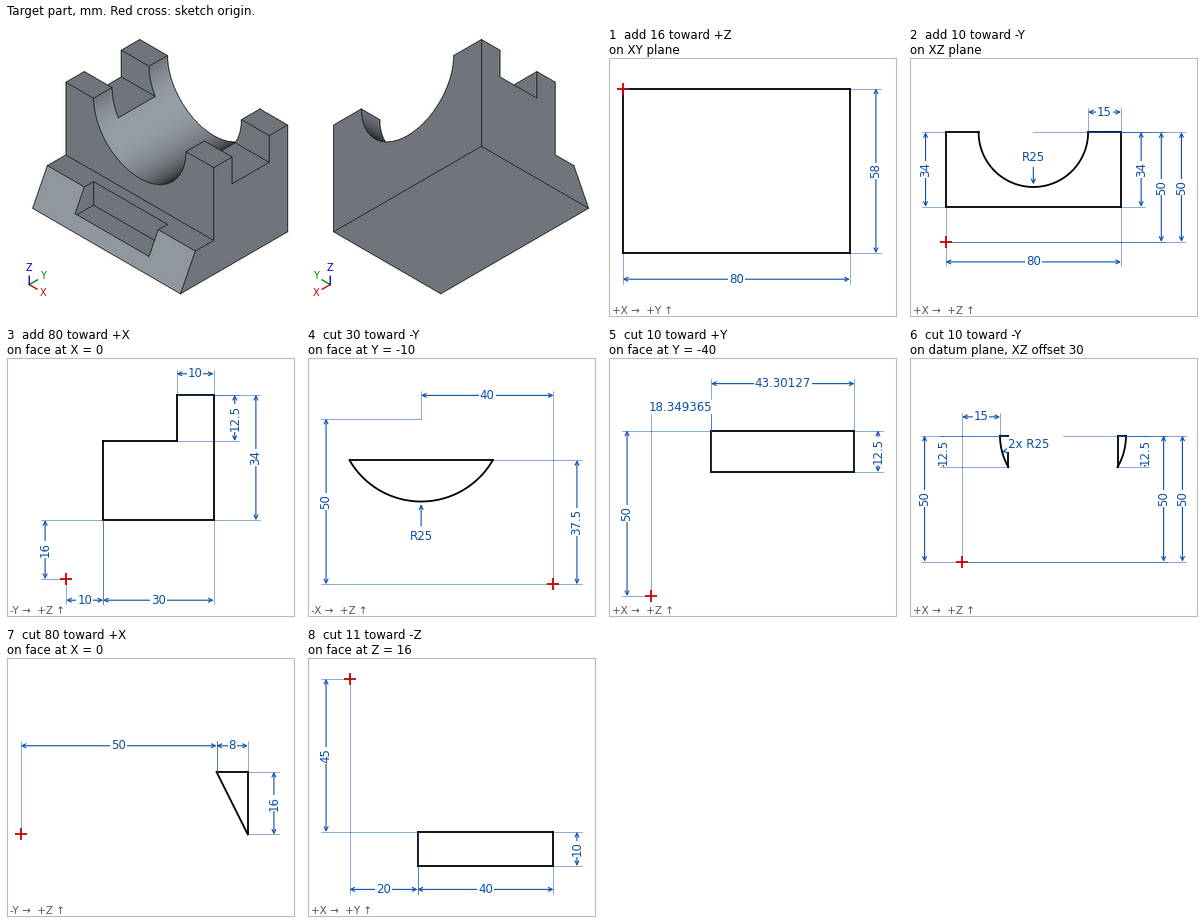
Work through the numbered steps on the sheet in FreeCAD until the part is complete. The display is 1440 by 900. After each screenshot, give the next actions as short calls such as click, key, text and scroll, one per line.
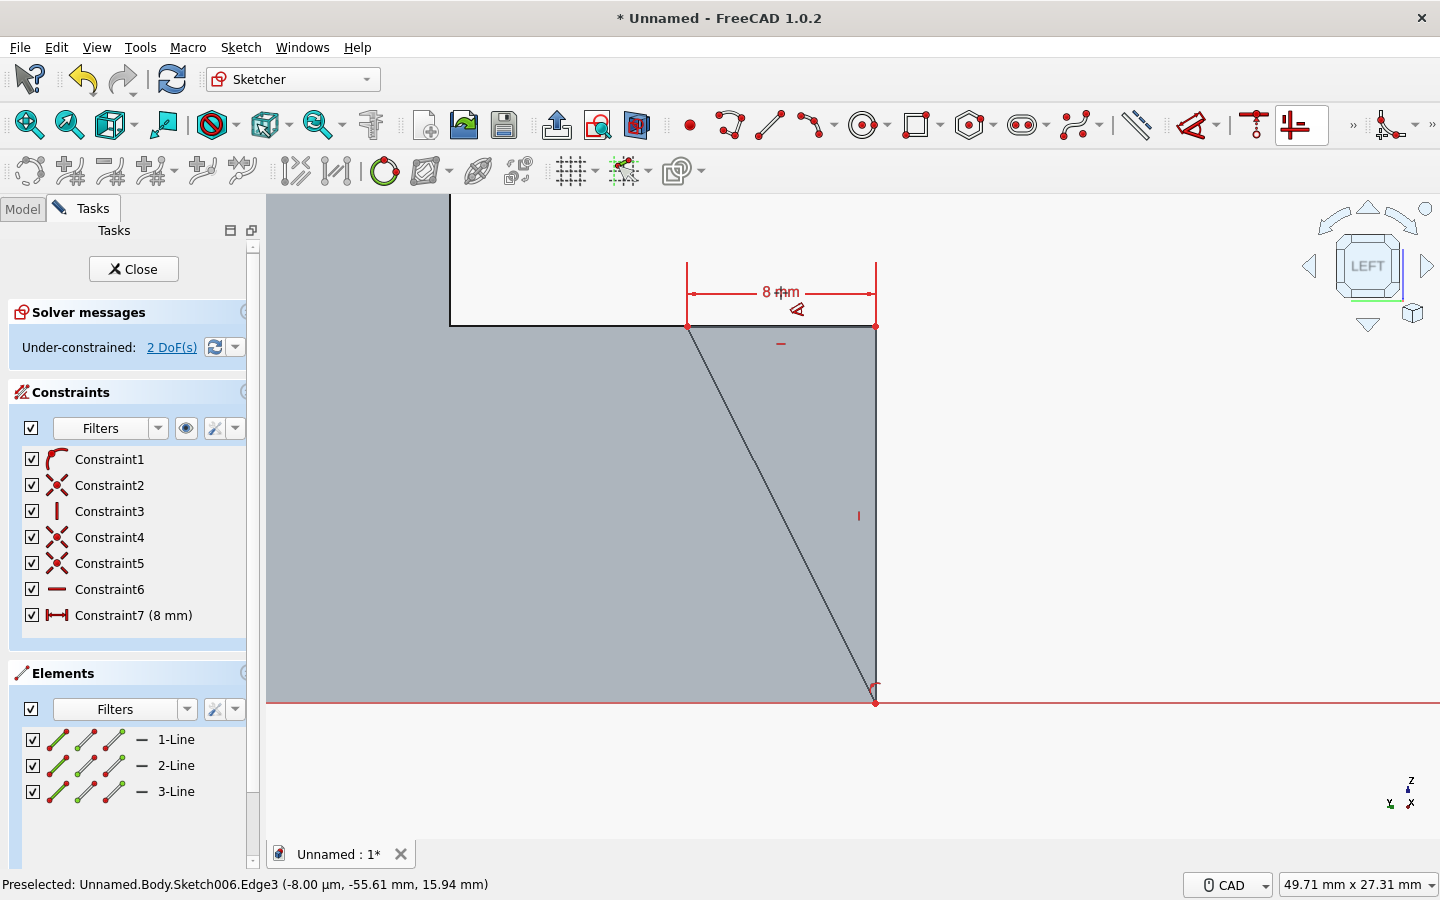
click(876, 591)
click(910, 515)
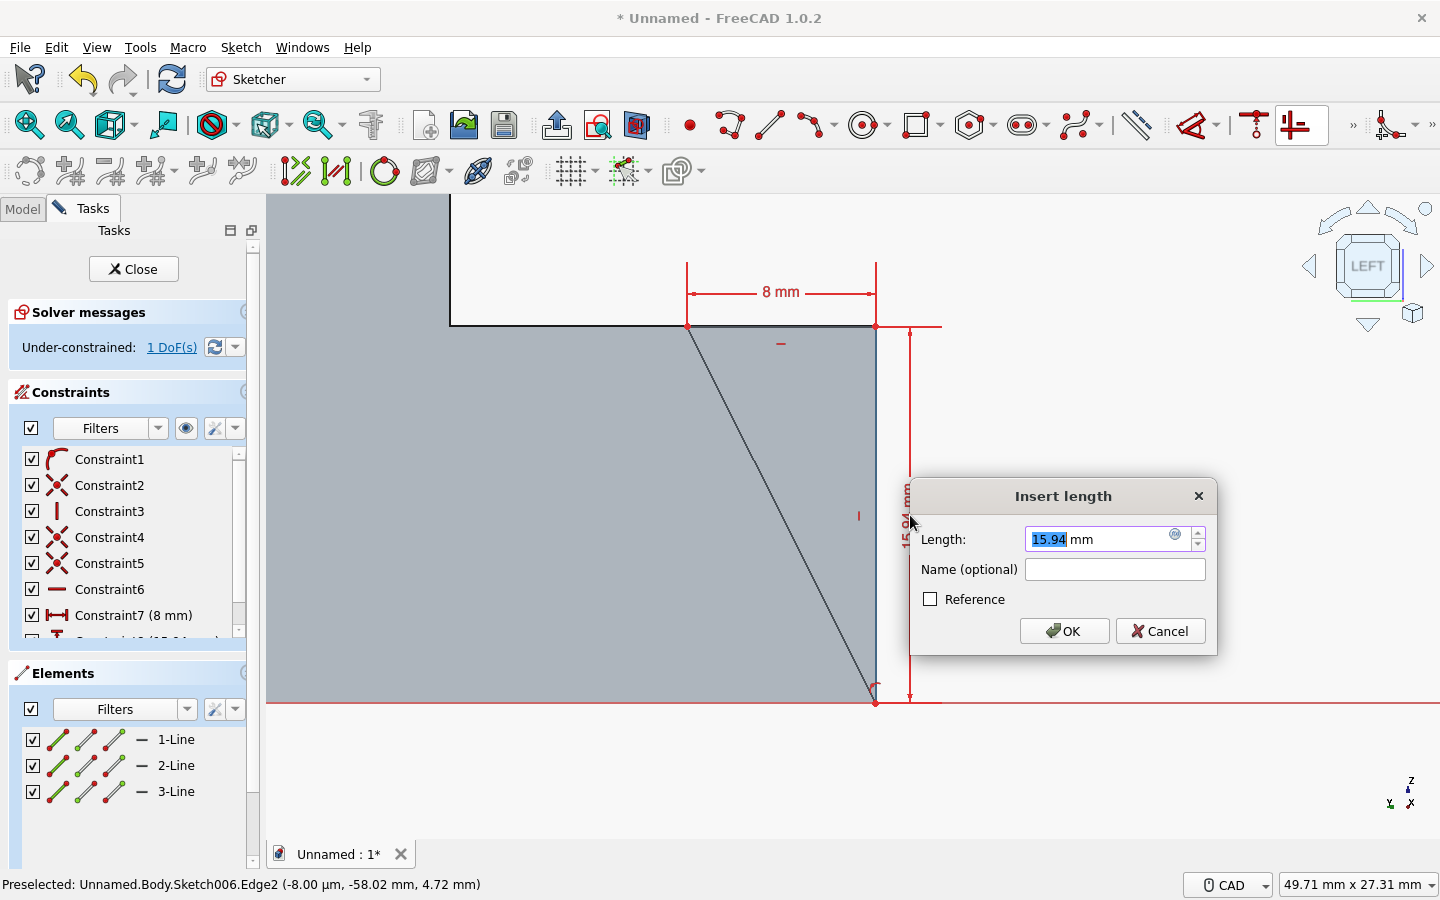
text(16)
key(Return)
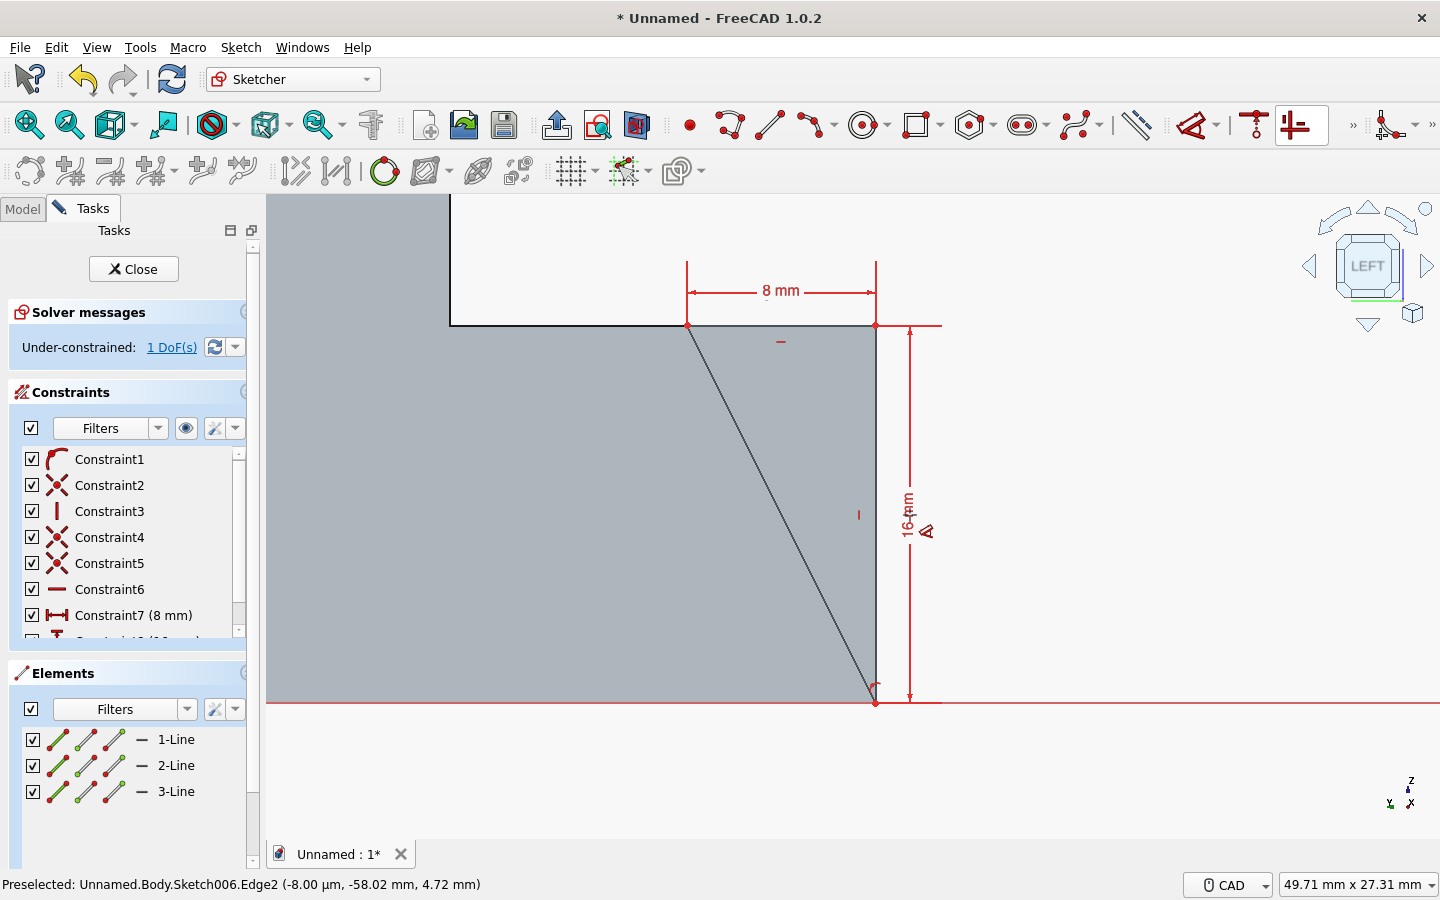
click(687, 326)
click(490, 737)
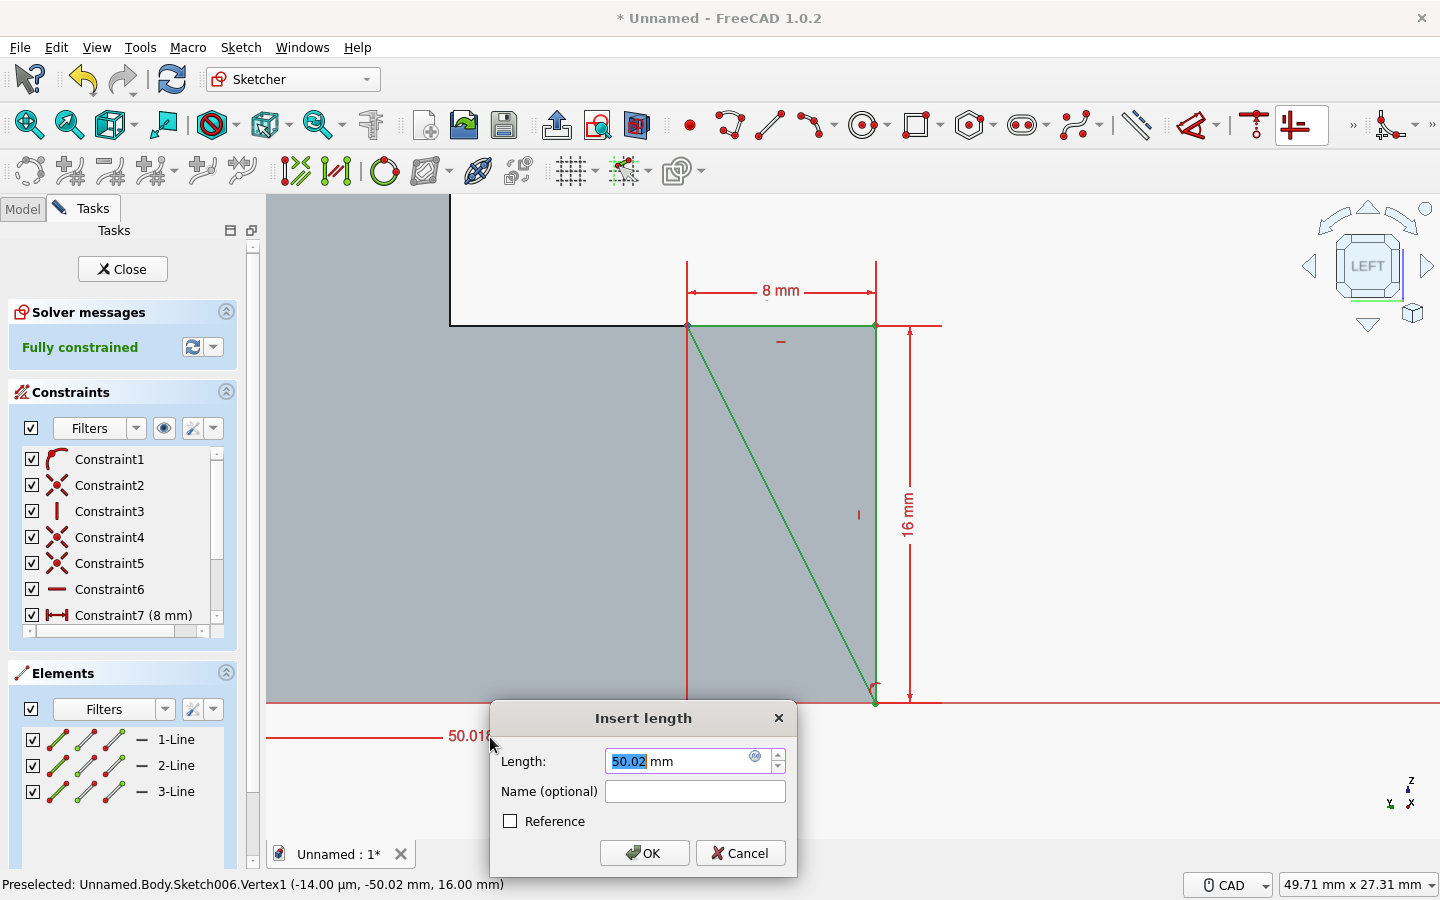
text(50)
key(Return)
key(Escape)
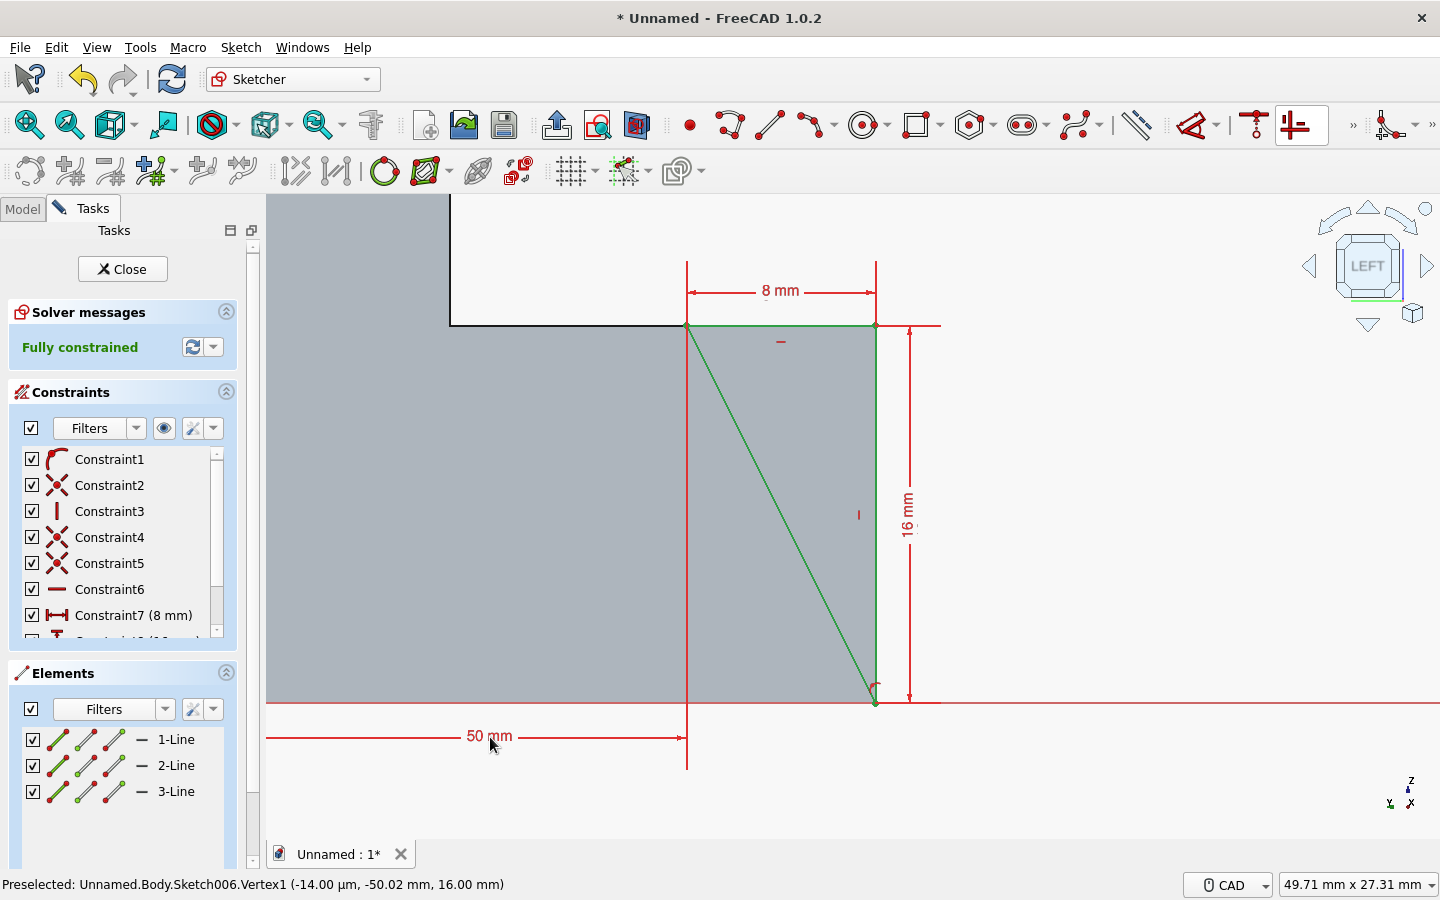
click(123, 269)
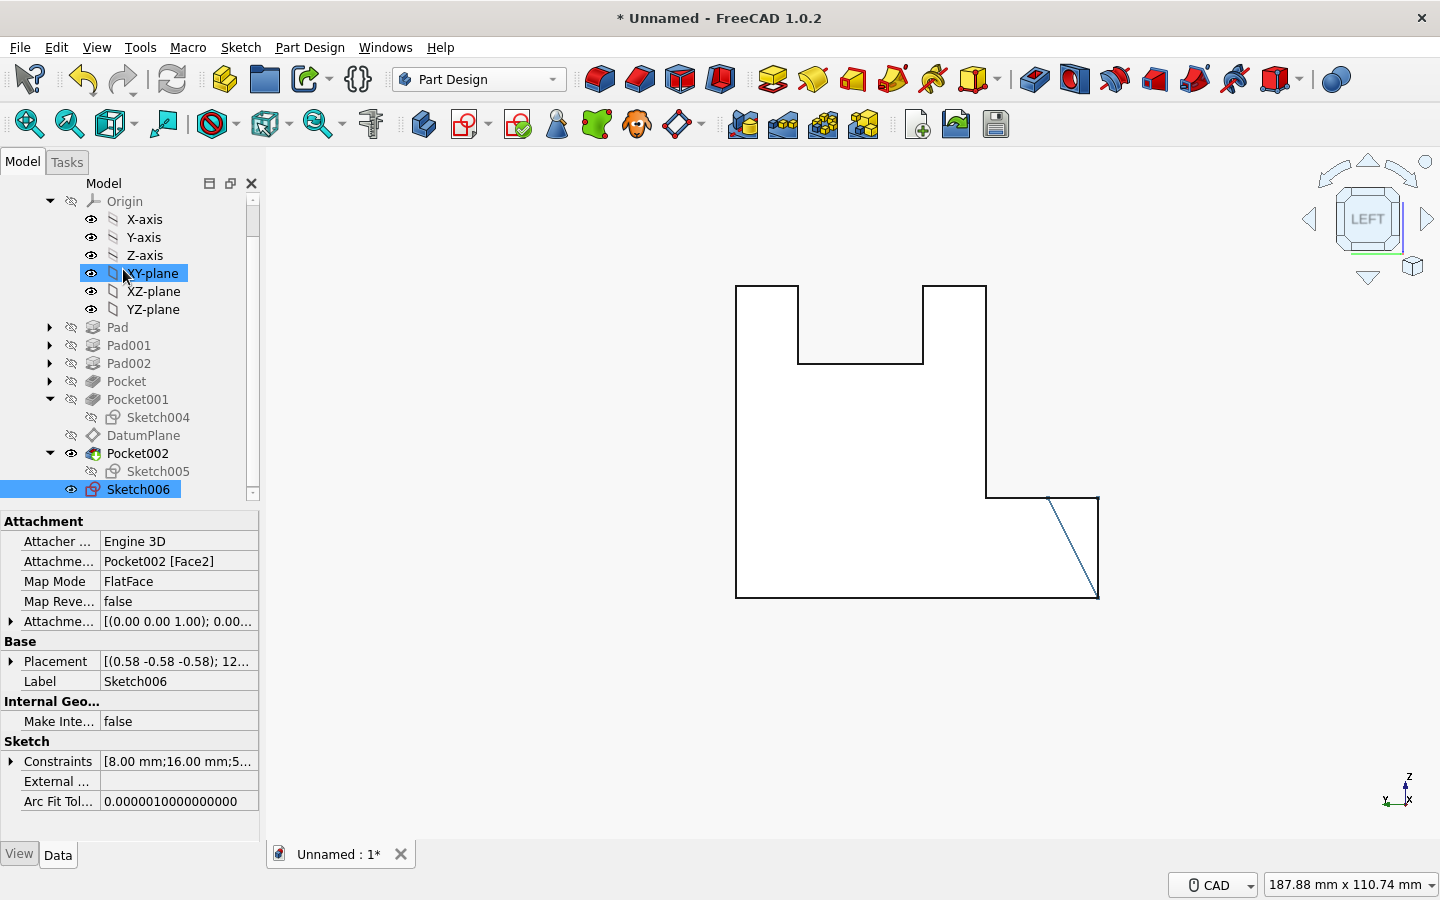
click(1036, 80)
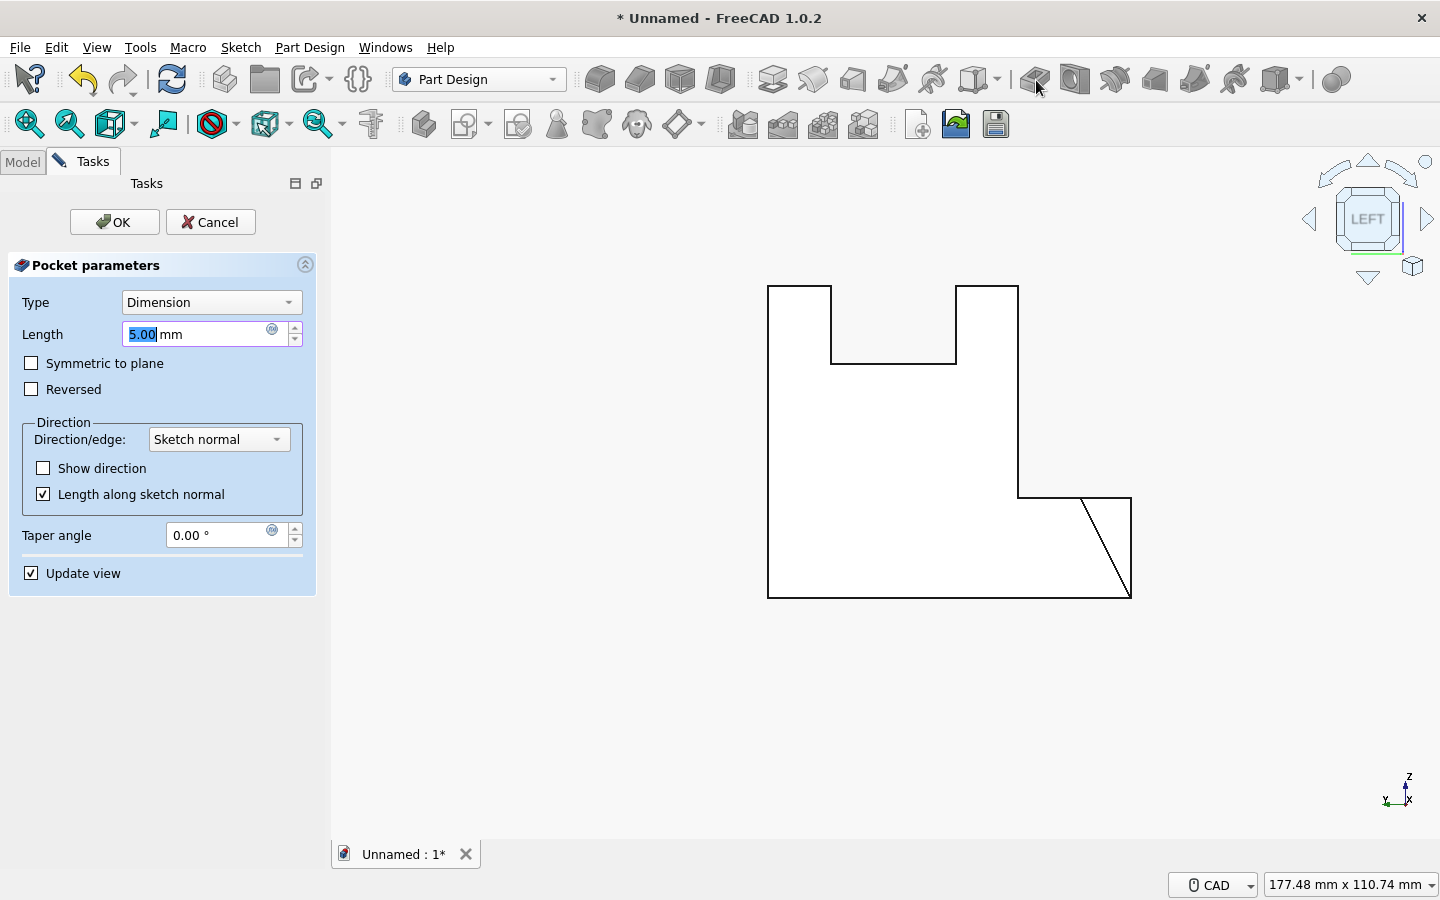
text(80)
key(Tab)